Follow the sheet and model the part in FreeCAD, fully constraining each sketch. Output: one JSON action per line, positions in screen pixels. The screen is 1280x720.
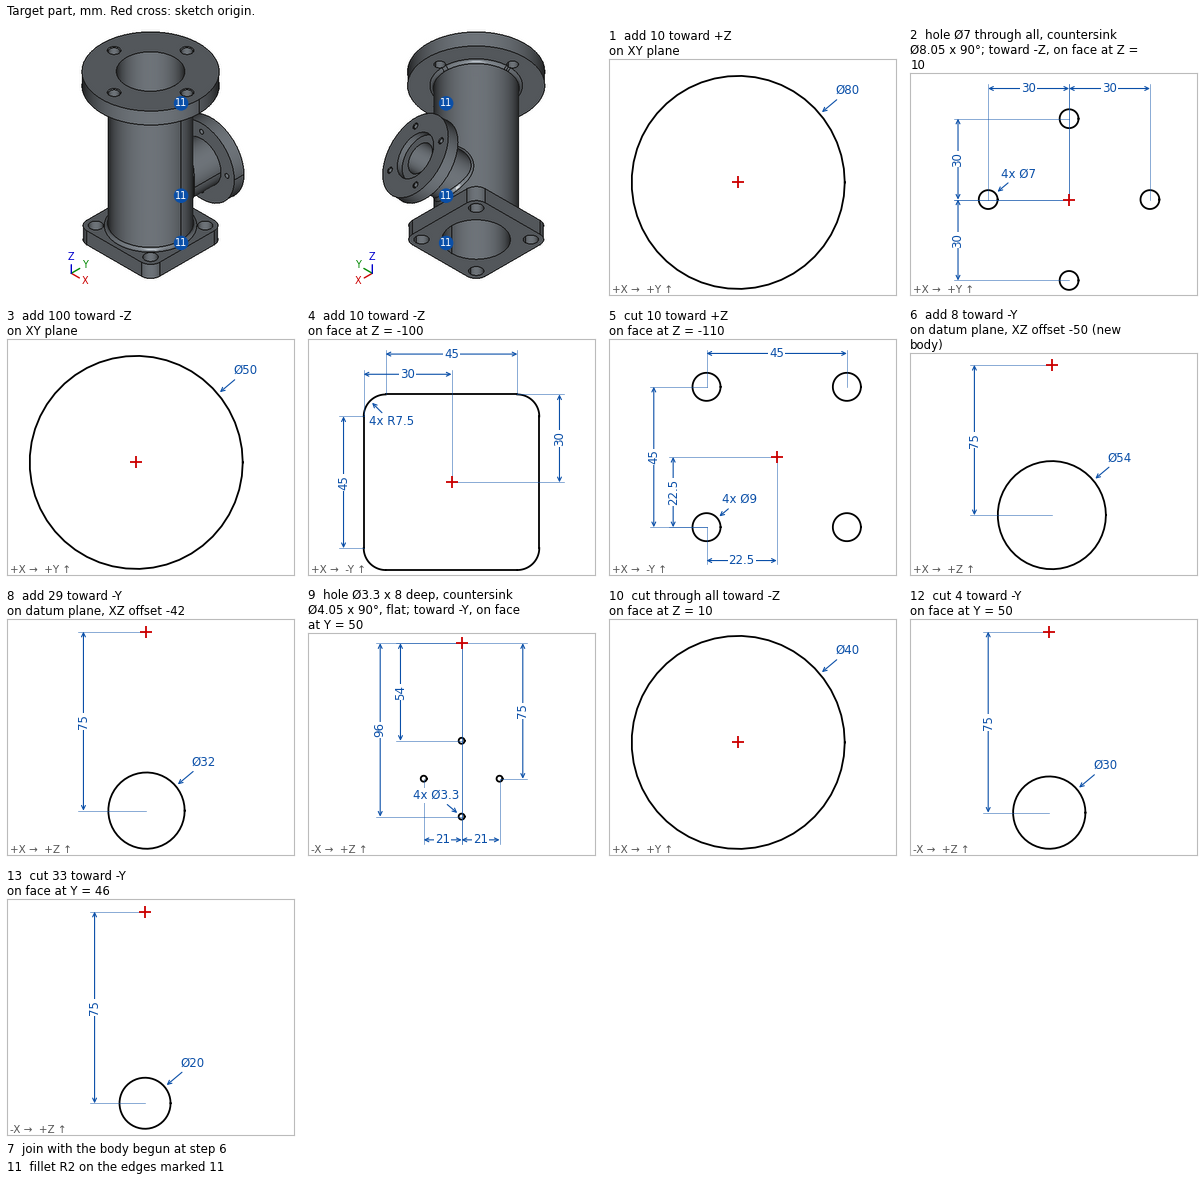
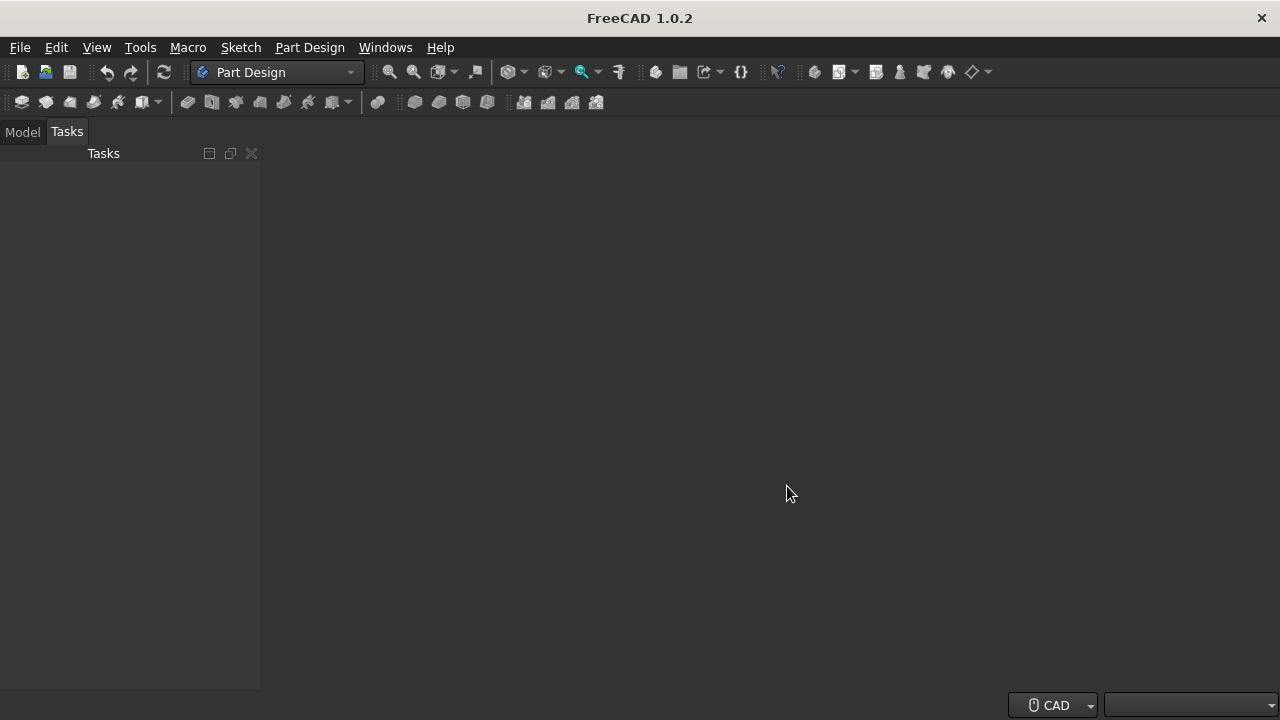
{"action": "left_click", "coordinate": [22, 72]}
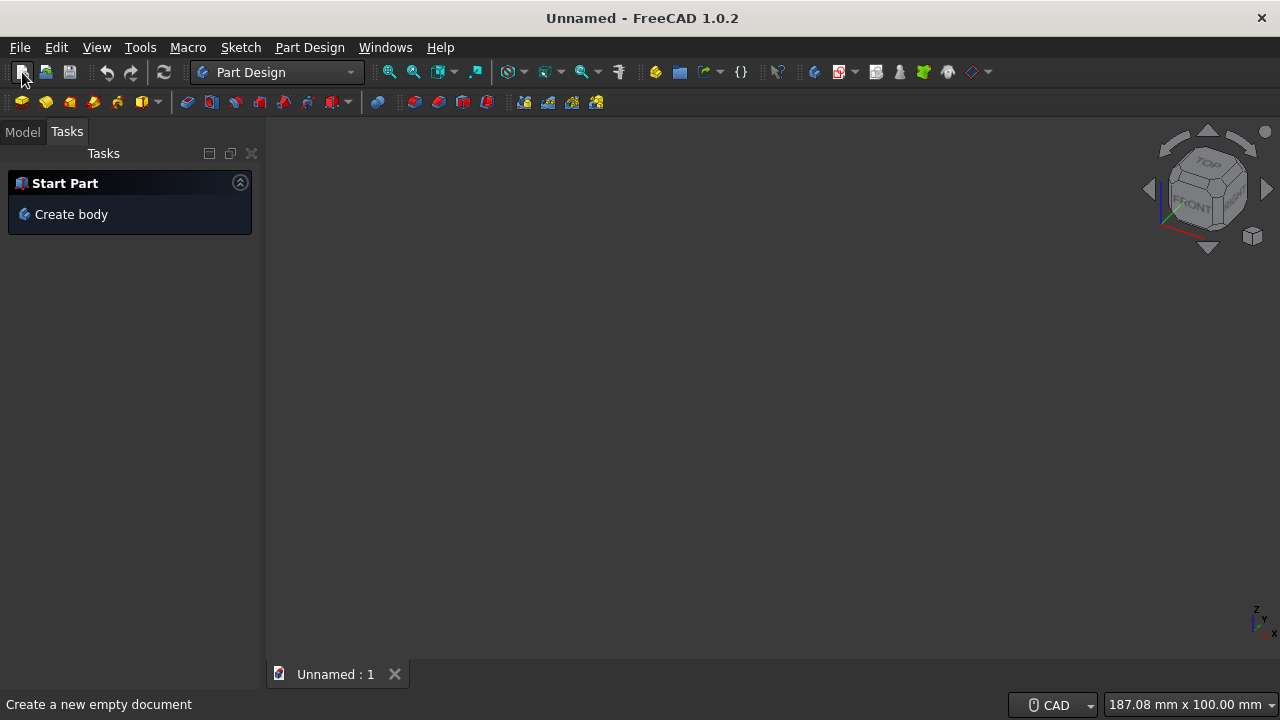
{"action": "left_click", "coordinate": [840, 72]}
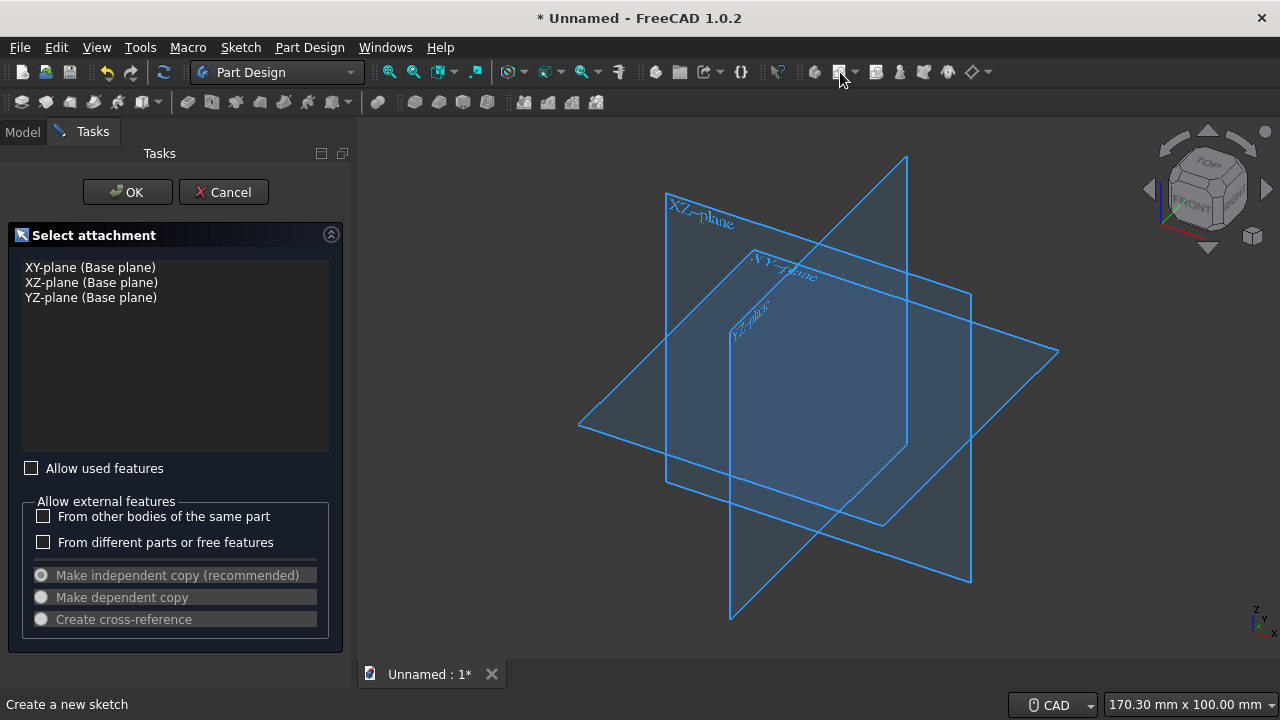
{"action": "left_click", "coordinate": [82, 268]}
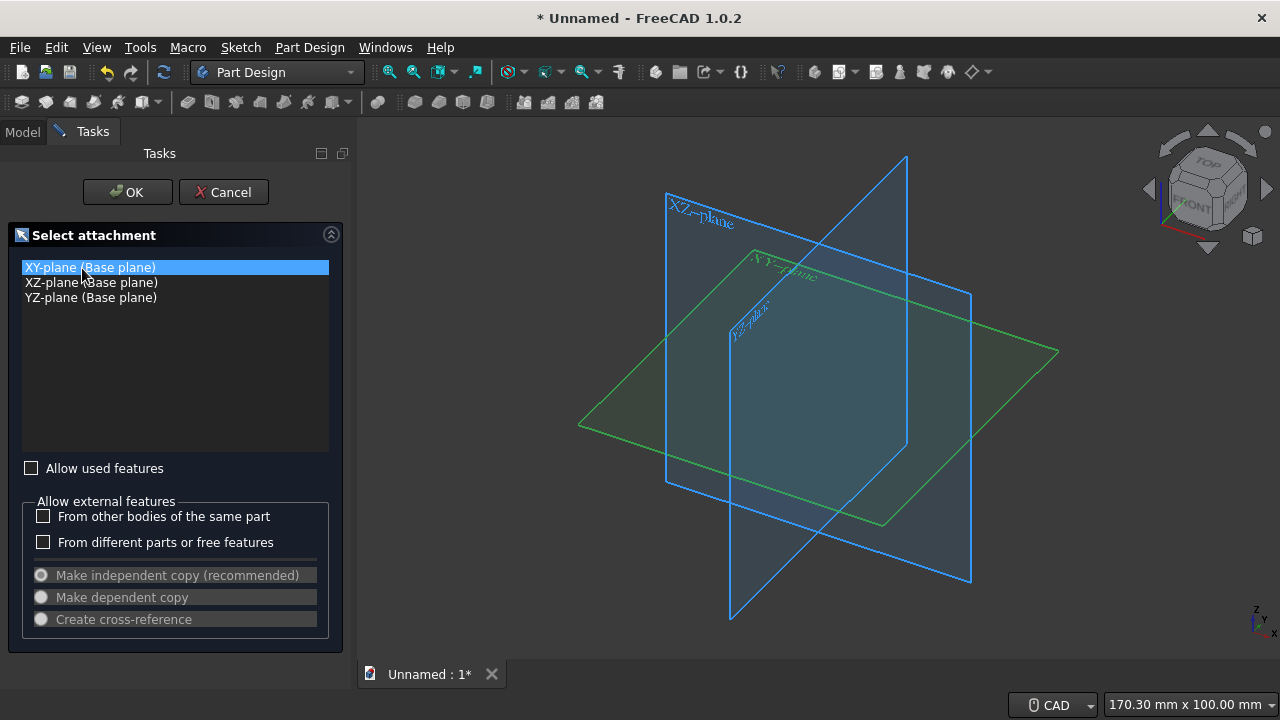
{"action": "left_click", "coordinate": [128, 192]}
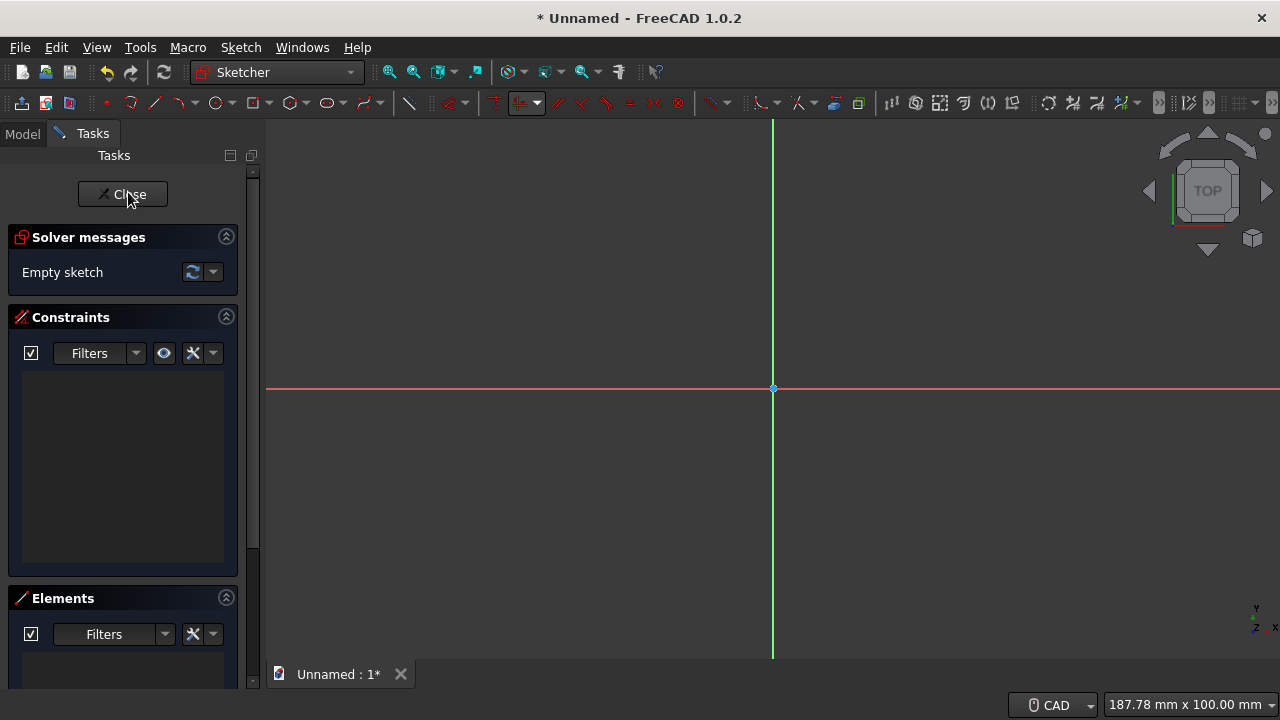
{"action": "left_click", "coordinate": [216, 104]}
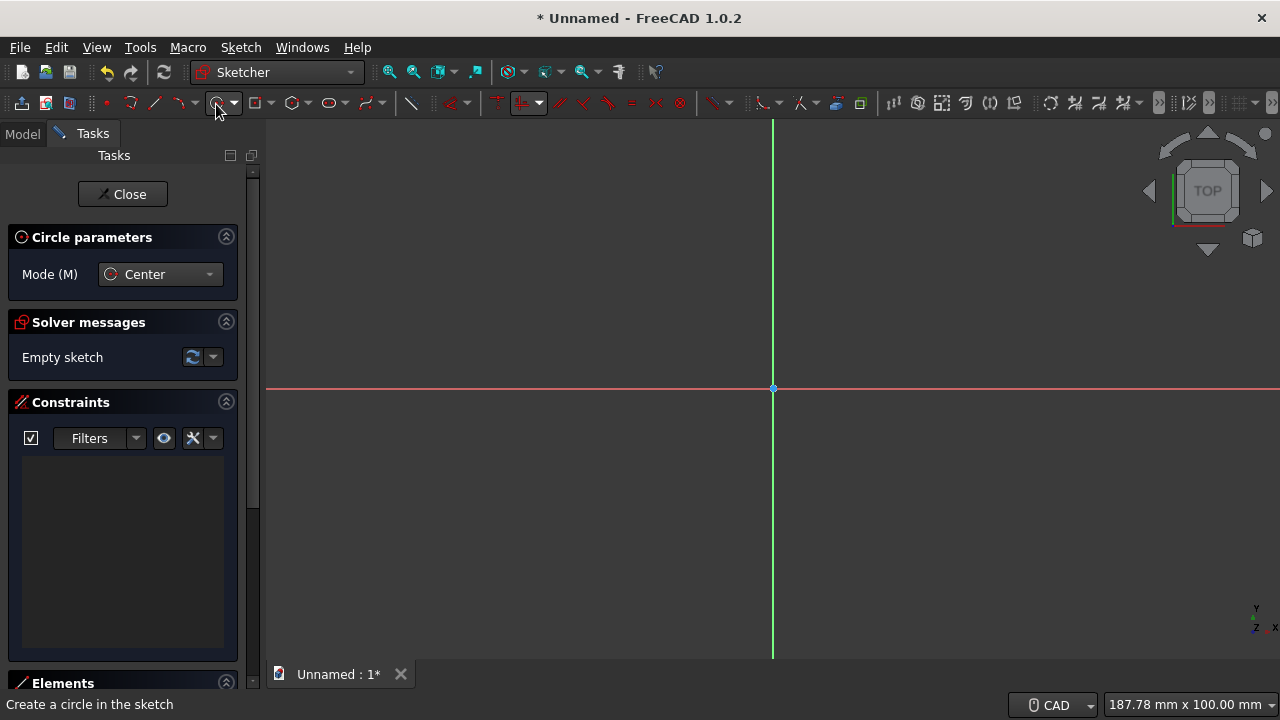
{"action": "left_click", "coordinate": [773, 389]}
{"action": "mouse_move", "coordinate": [926, 236]}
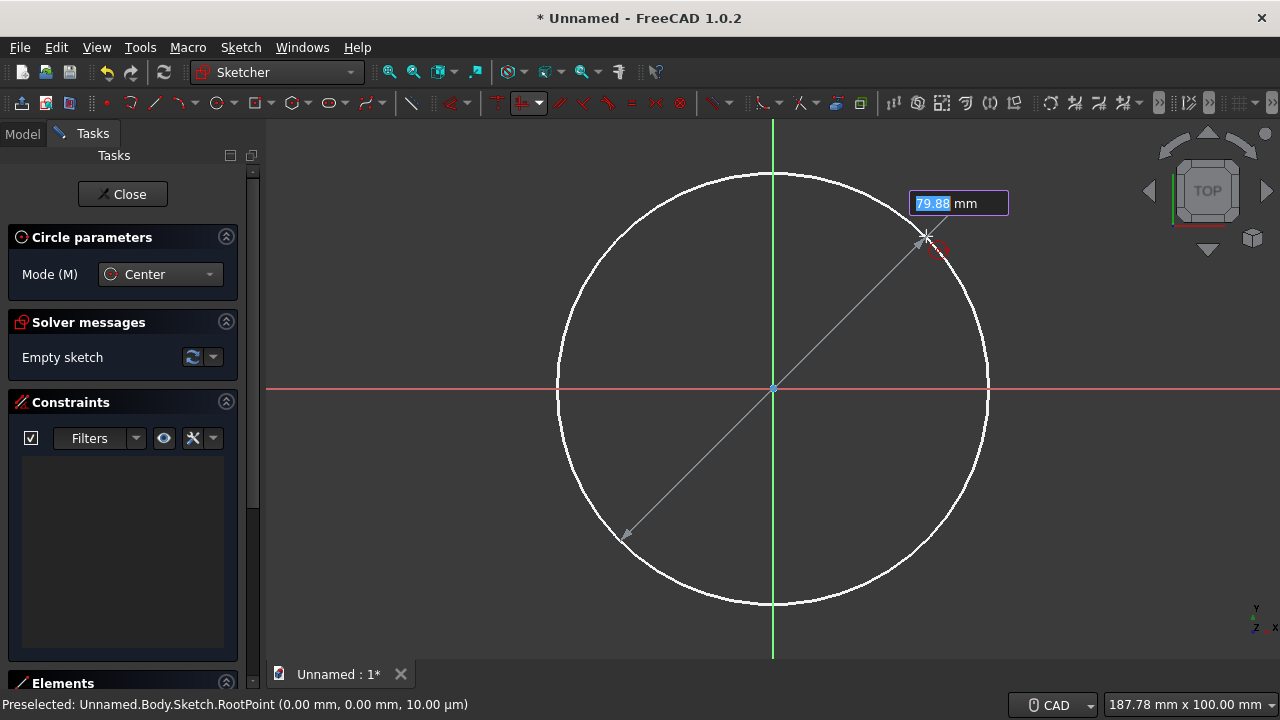
{"action": "type", "text": "80"}
{"action": "key", "text": "Return"}
{"action": "key", "text": "Escape"}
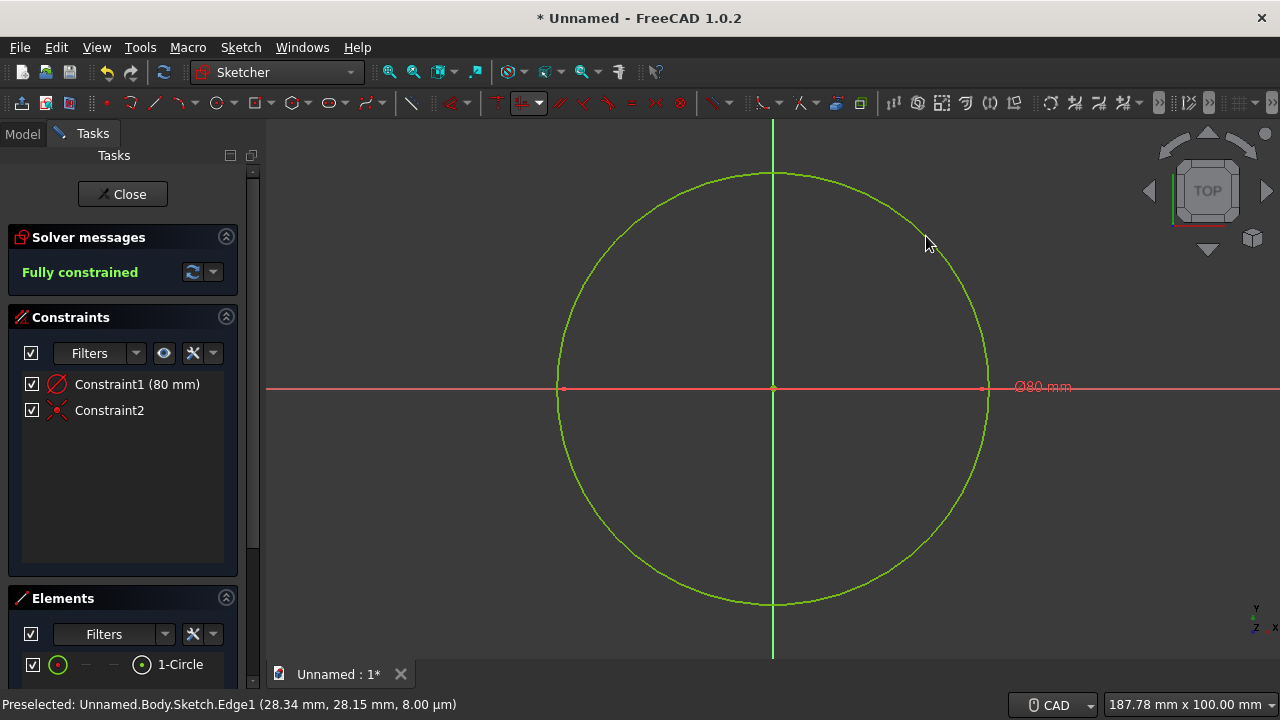
{"action": "left_click", "coordinate": [123, 194]}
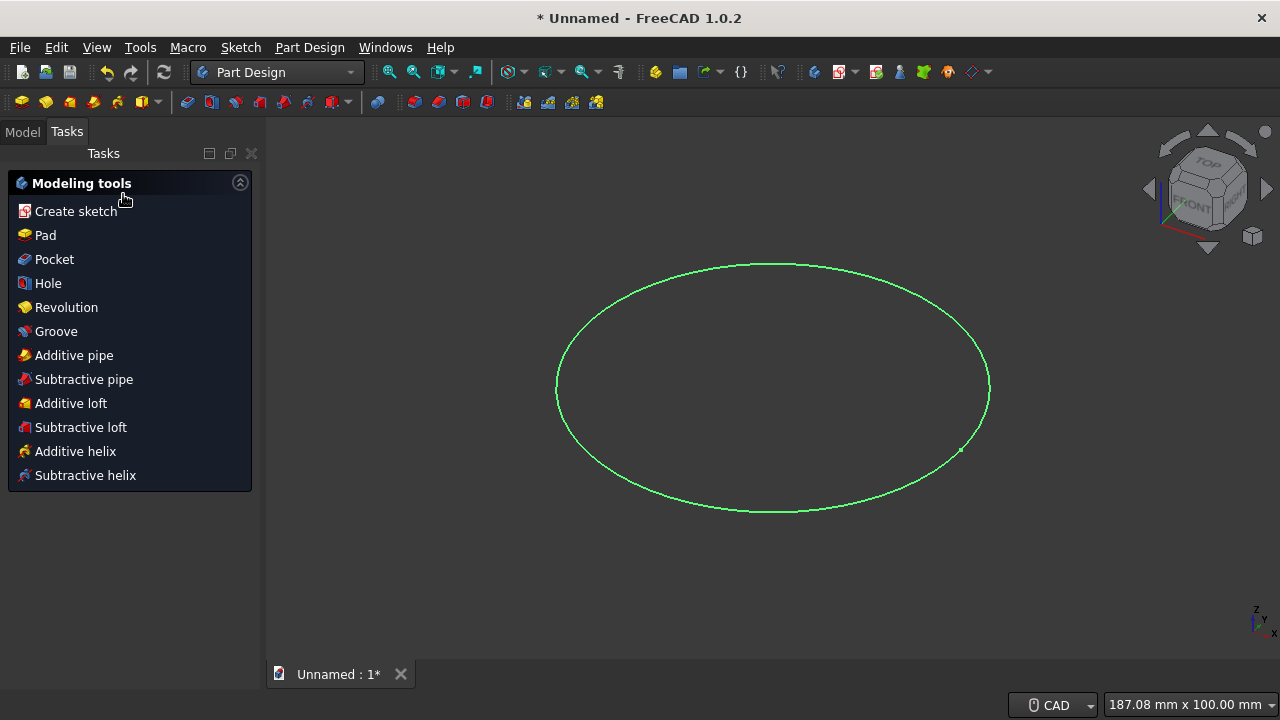
{"action": "left_click", "coordinate": [22, 102]}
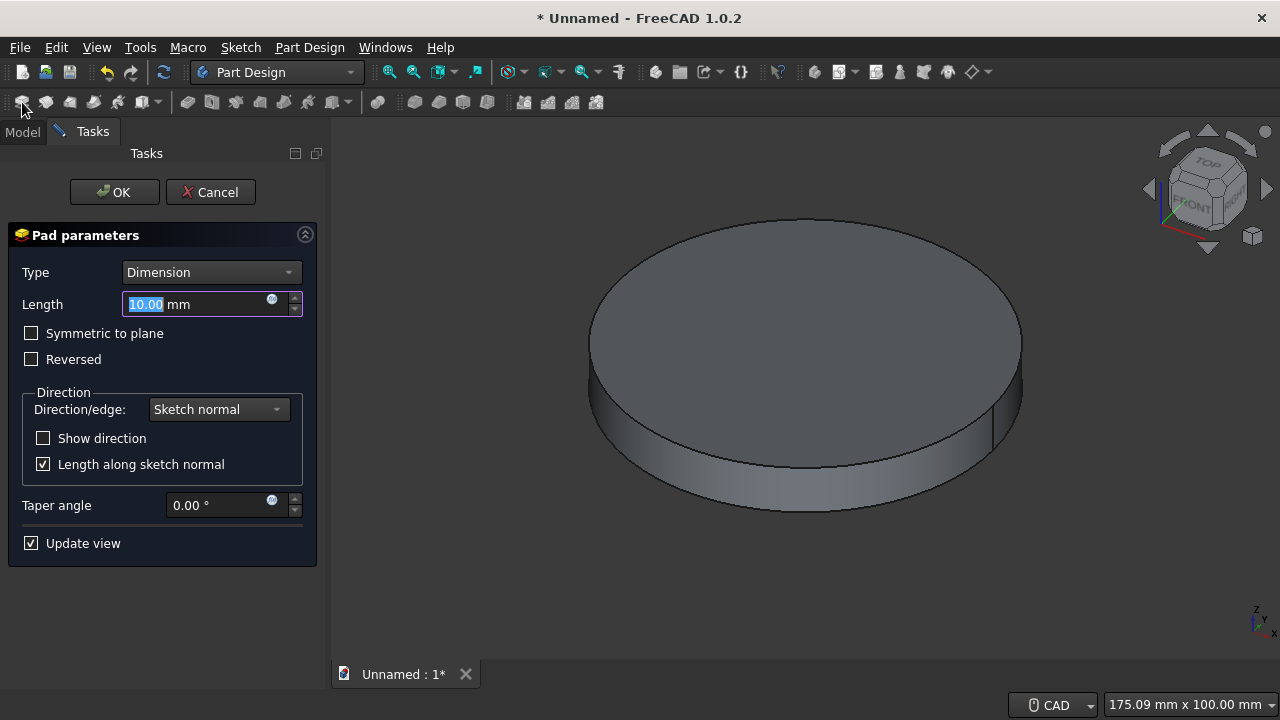
{"action": "type", "text": "10"}
{"action": "key", "text": "Tab"}